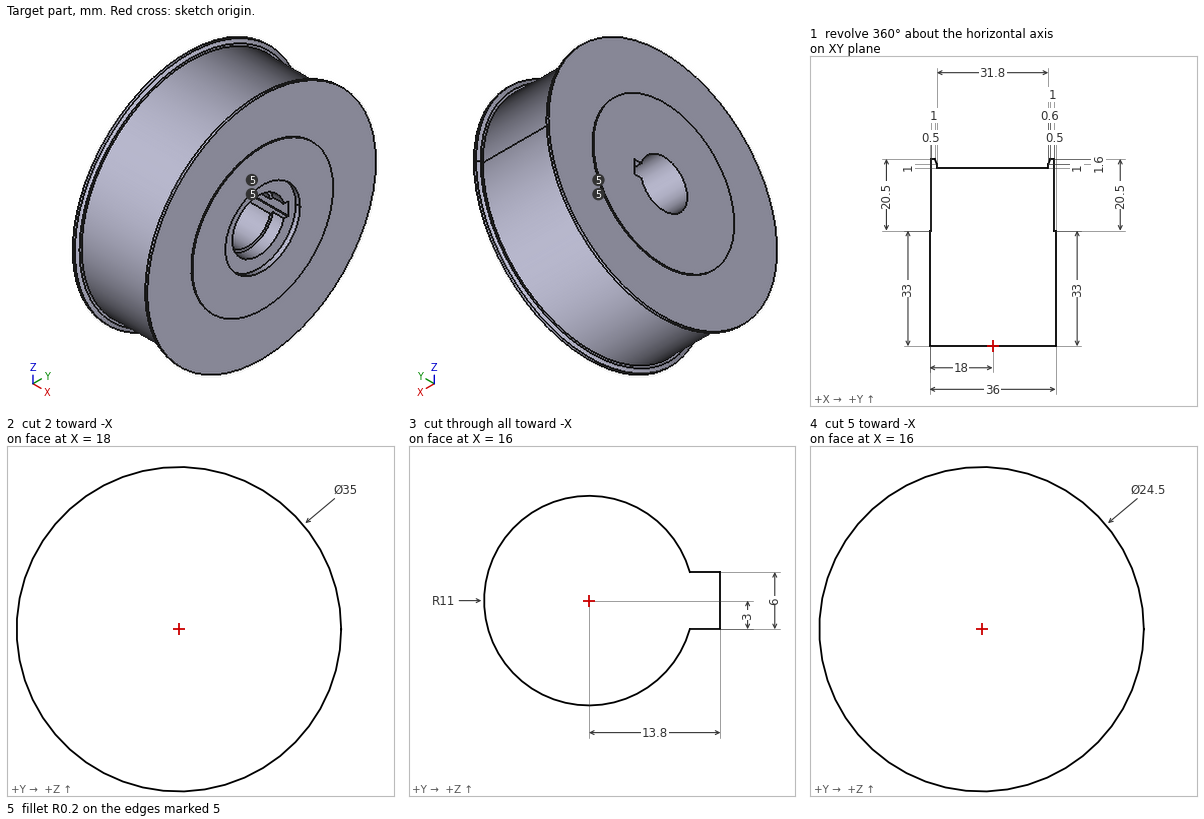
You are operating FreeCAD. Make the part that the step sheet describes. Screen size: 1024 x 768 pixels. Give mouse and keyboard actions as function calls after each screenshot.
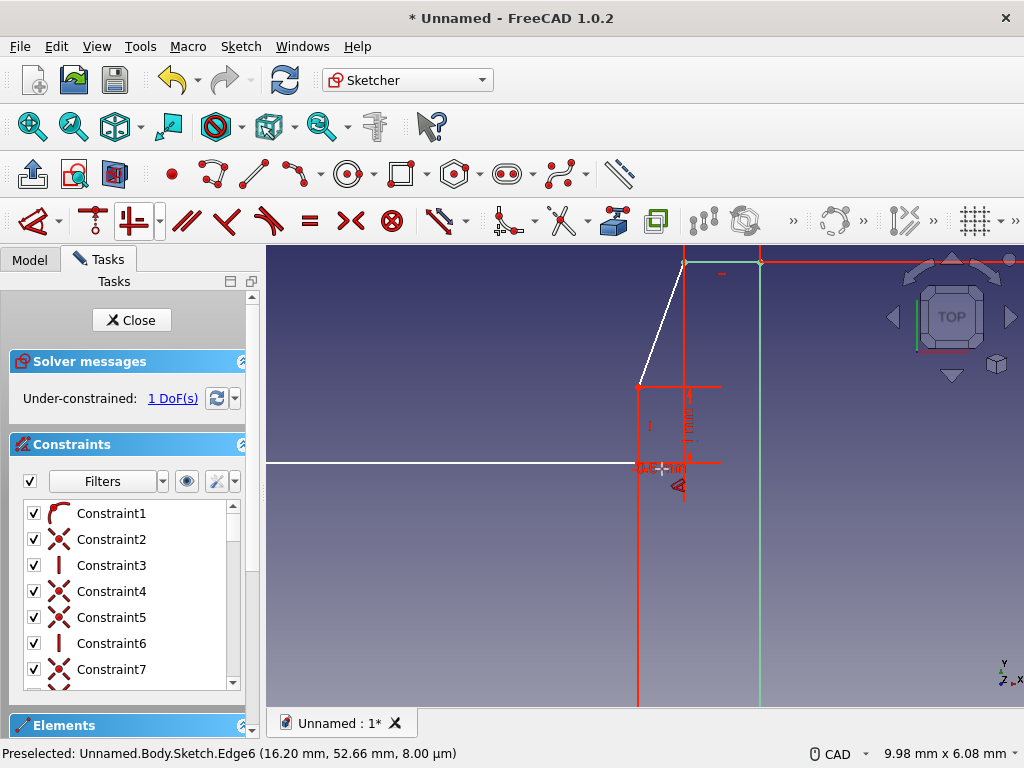
scroll(668, 330, down, 13)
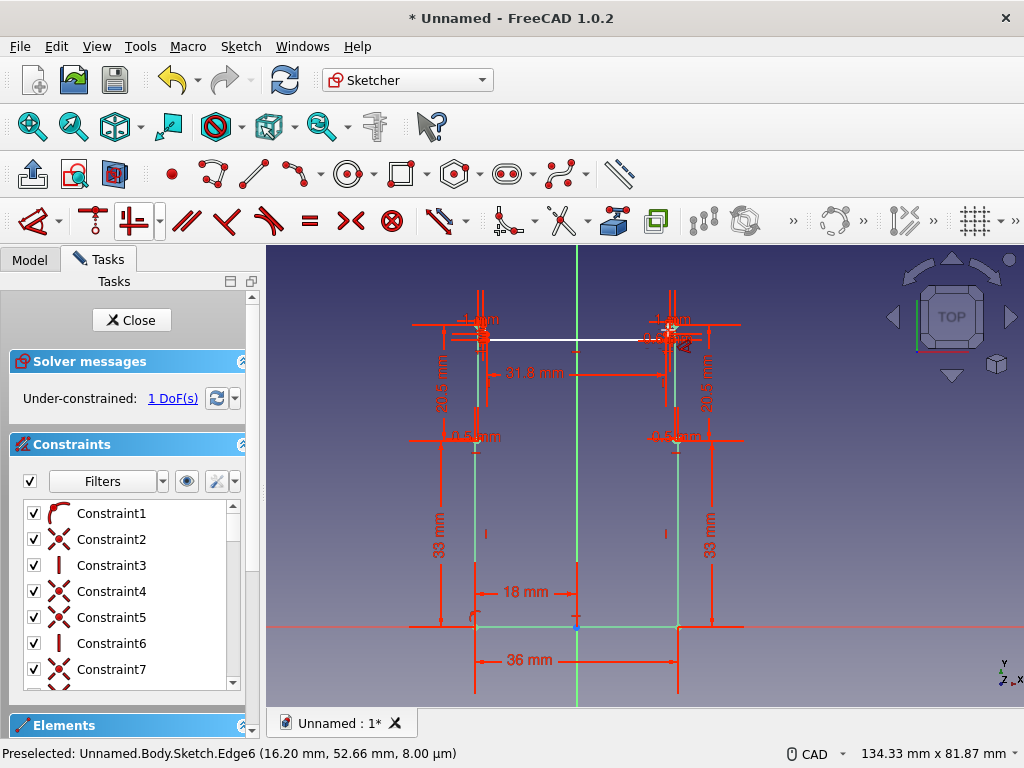
scroll(669, 328, up, 8)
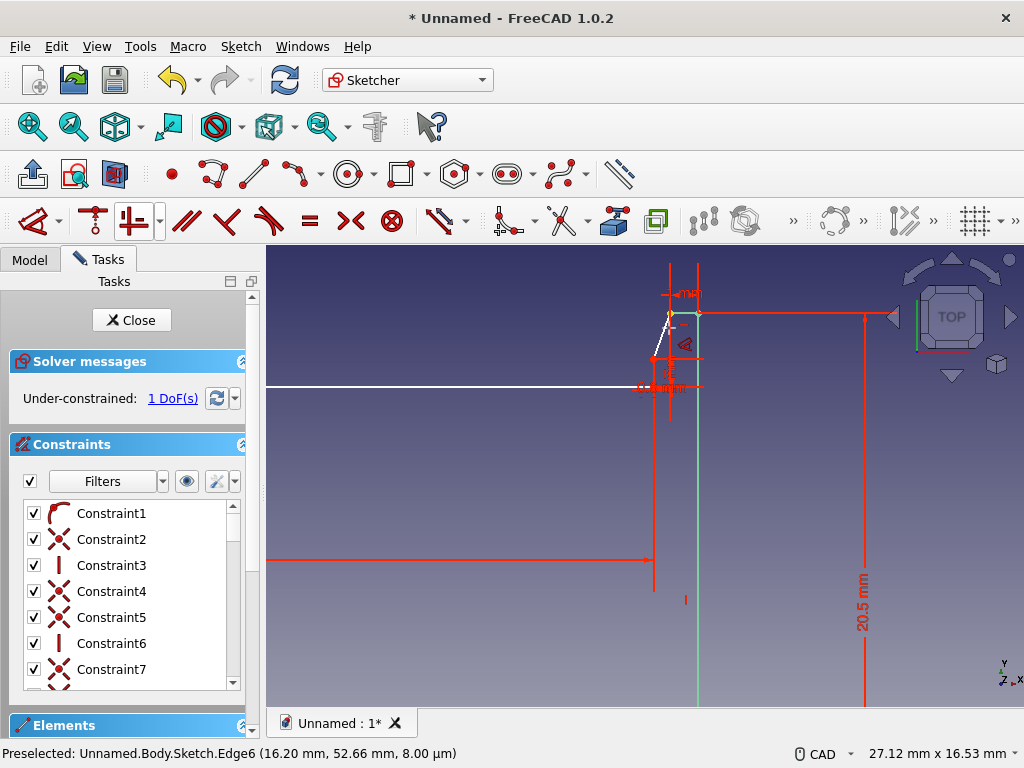
click(665, 327)
click(620, 336)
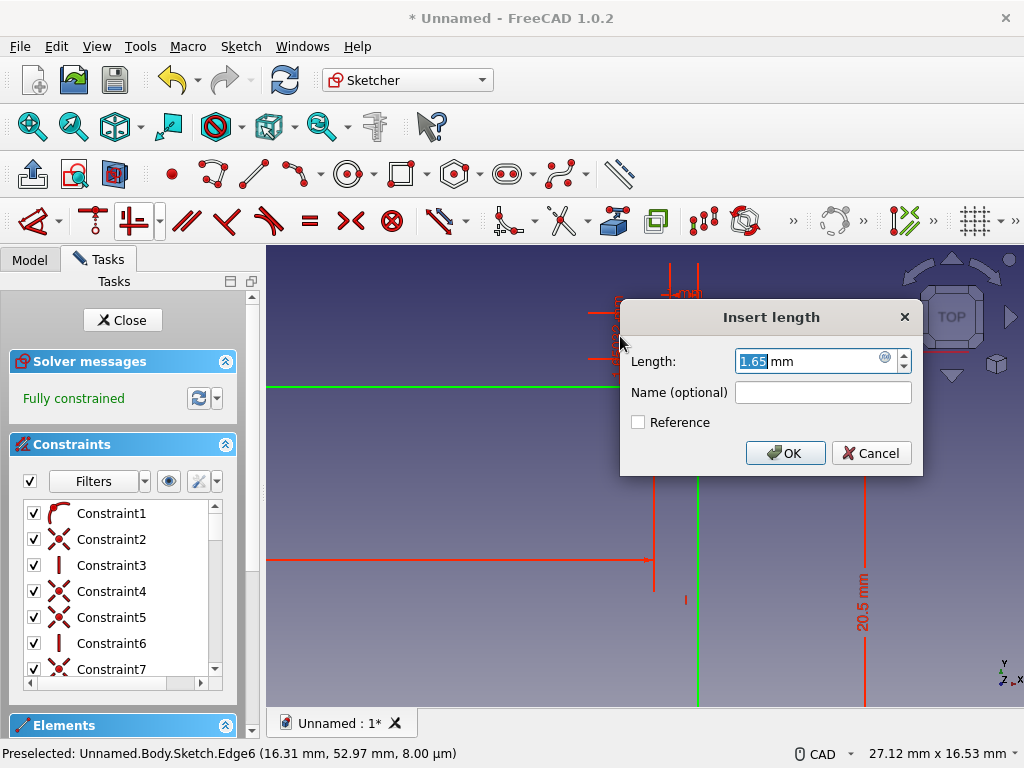
text(1.6)
key(Return)
key(Escape)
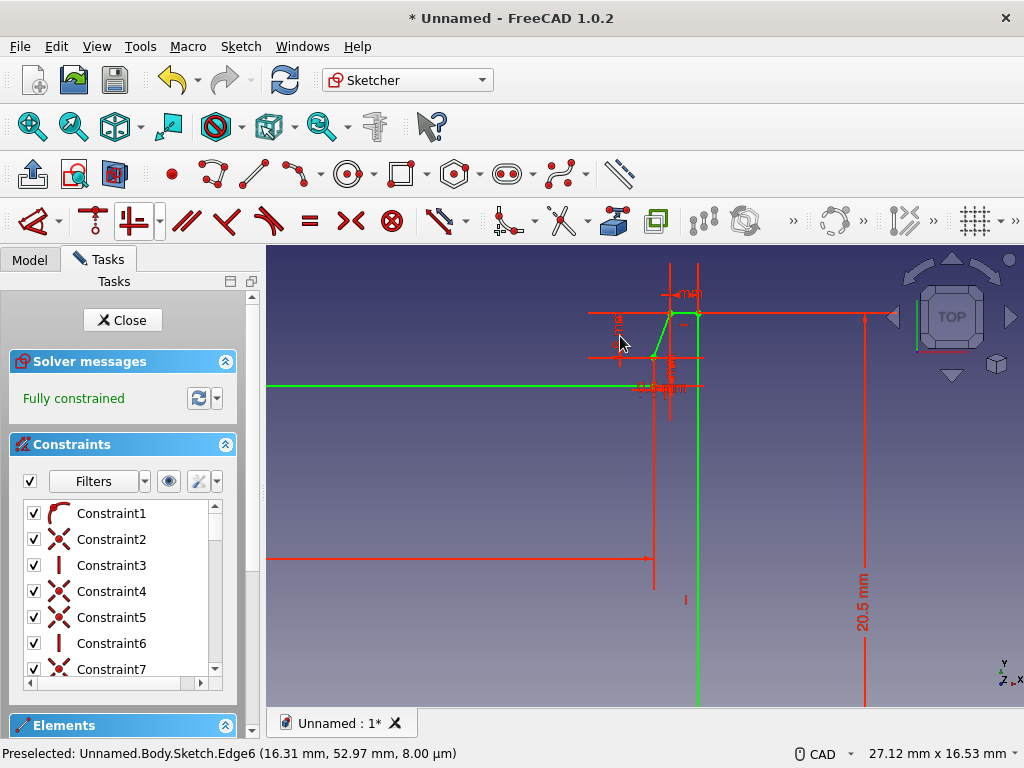
click(123, 320)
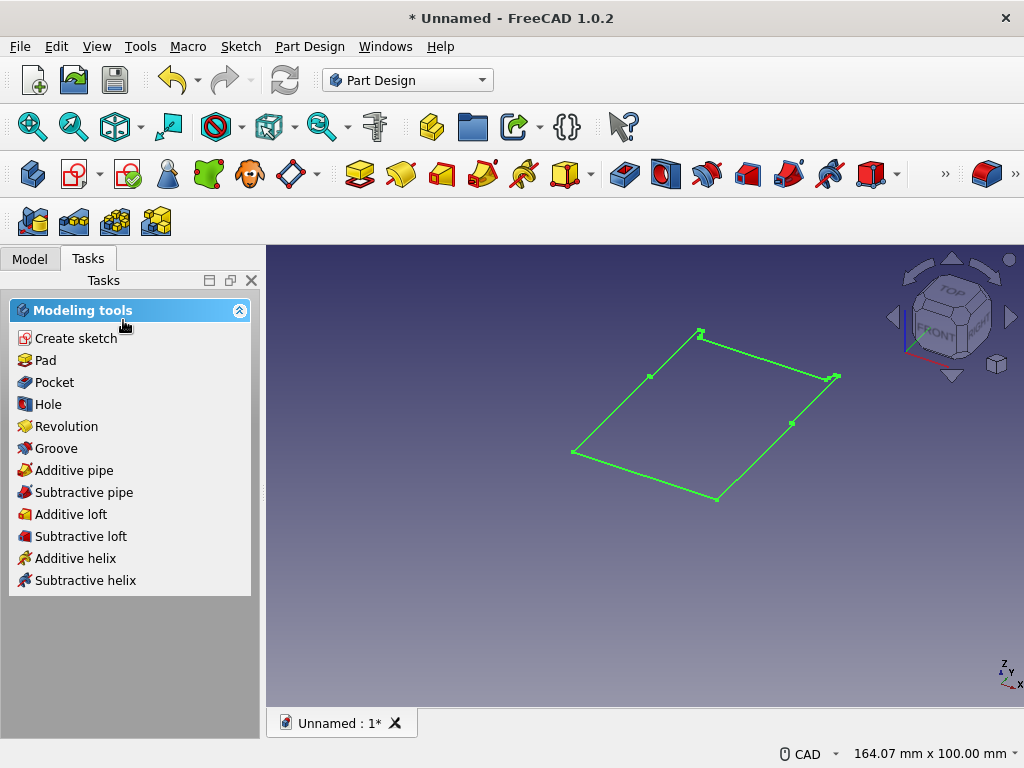
click(401, 174)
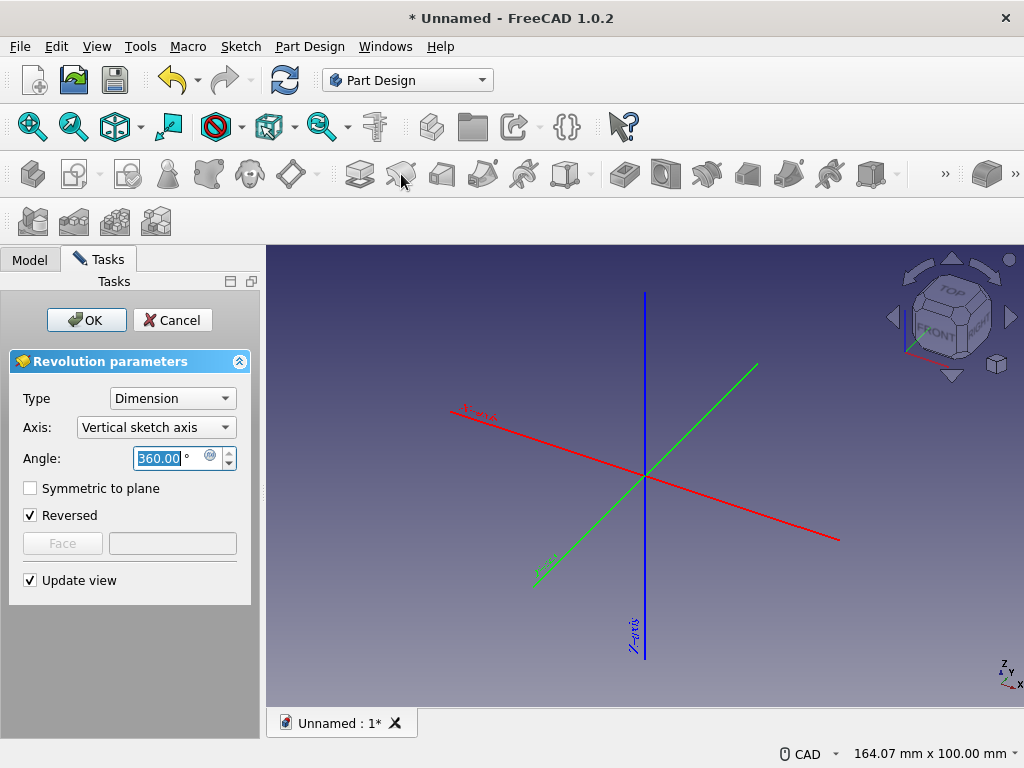
click(157, 428)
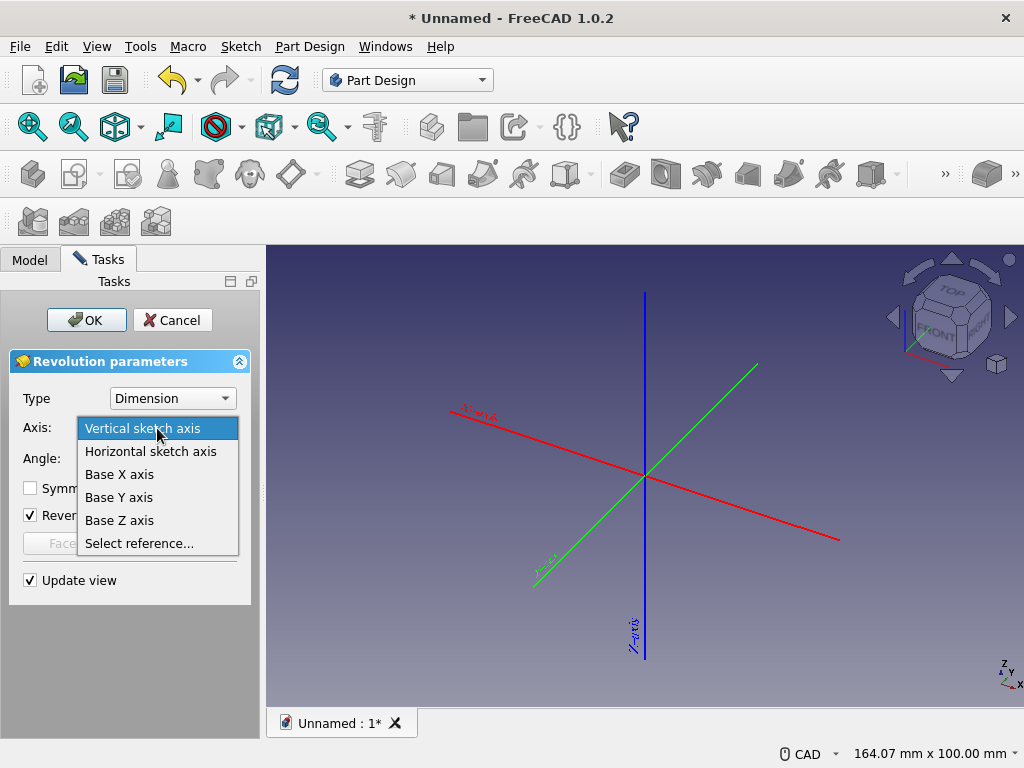
click(156, 452)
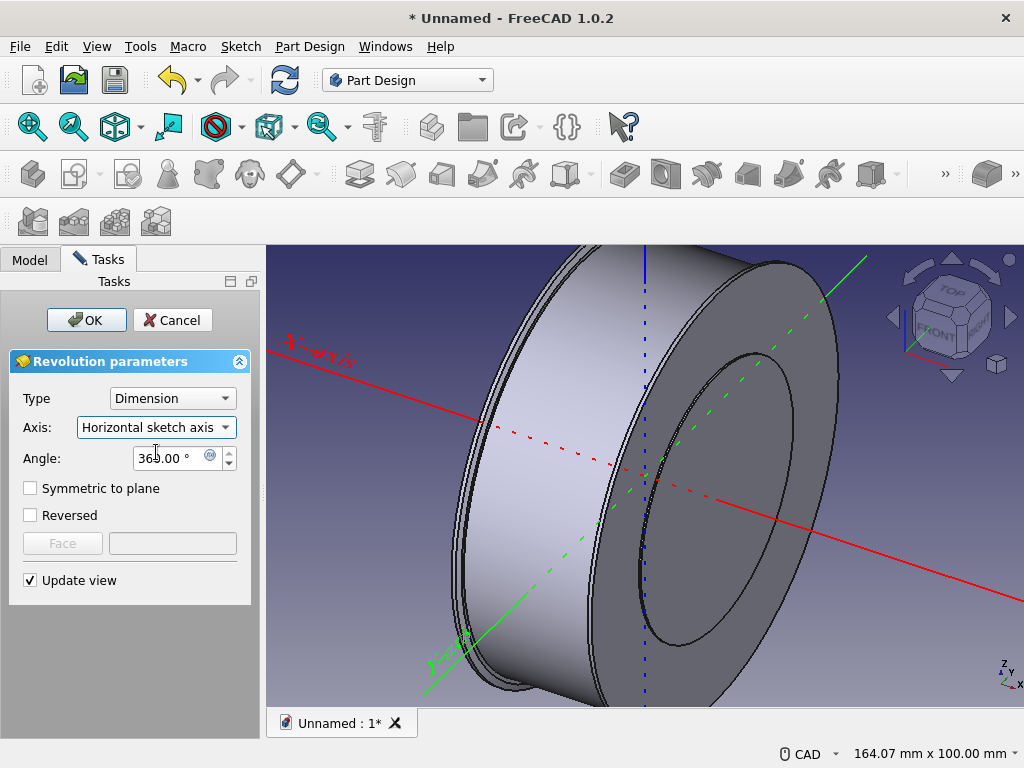
click(87, 320)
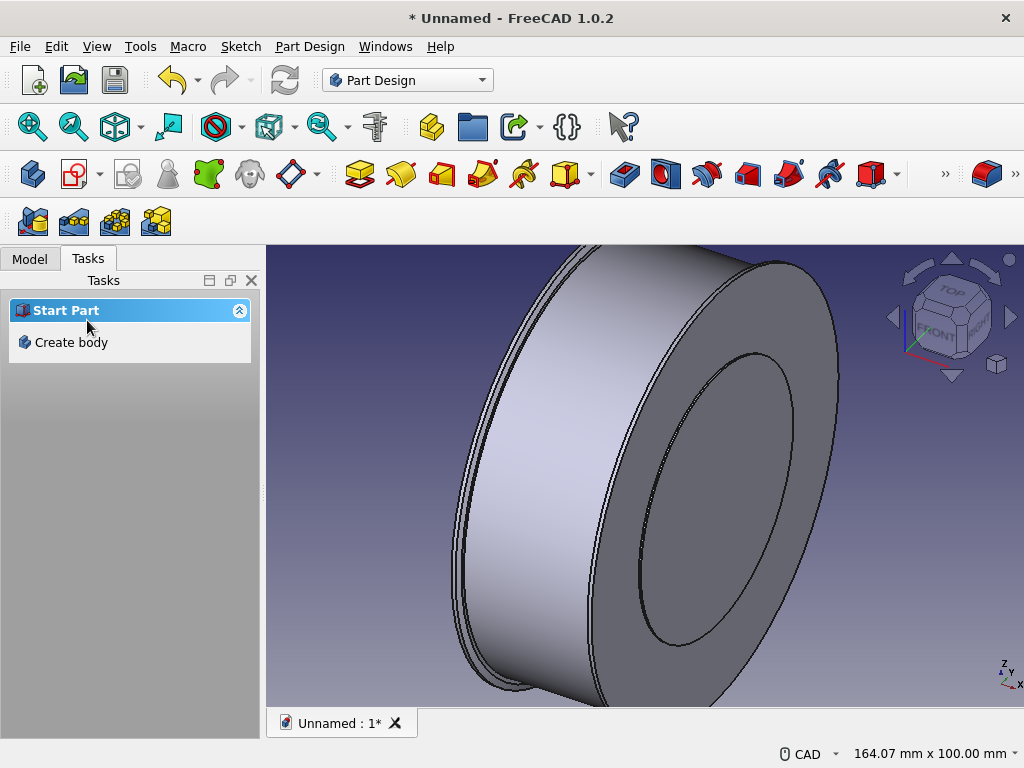
click(33, 128)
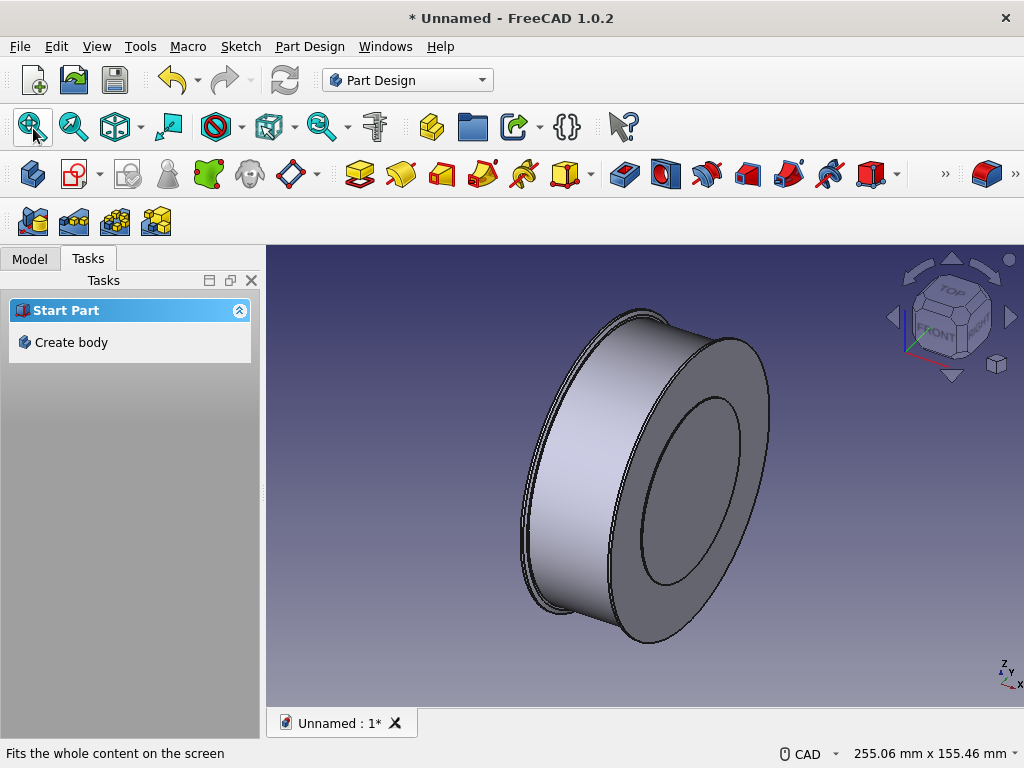
click(691, 490)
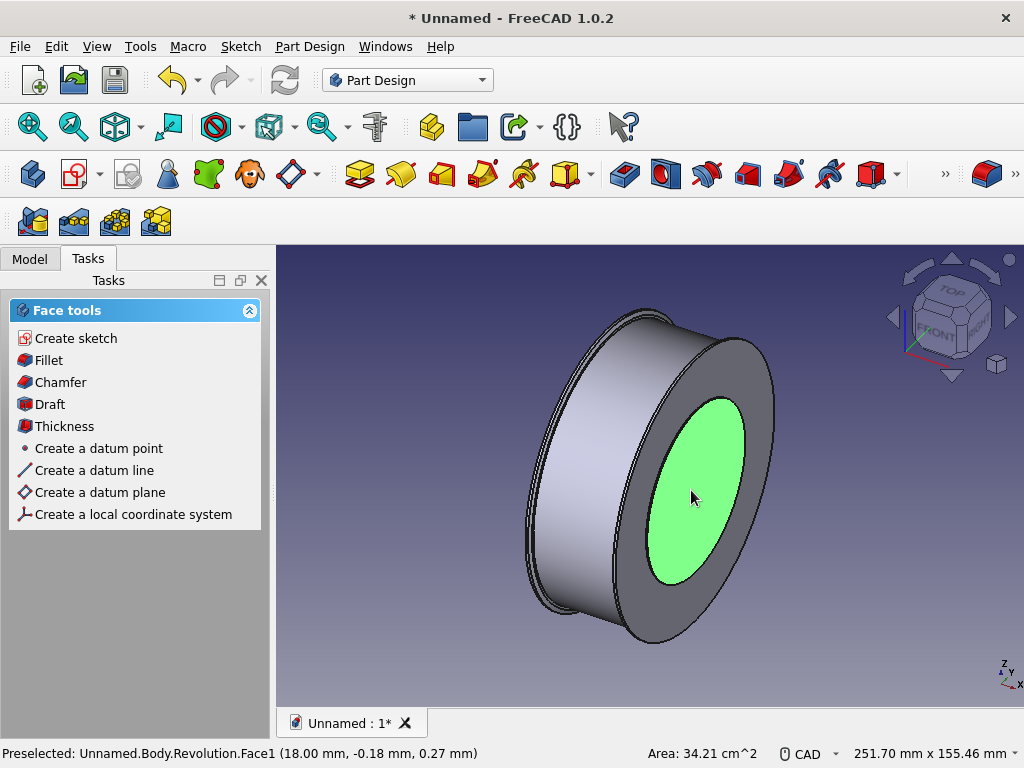
click(74, 174)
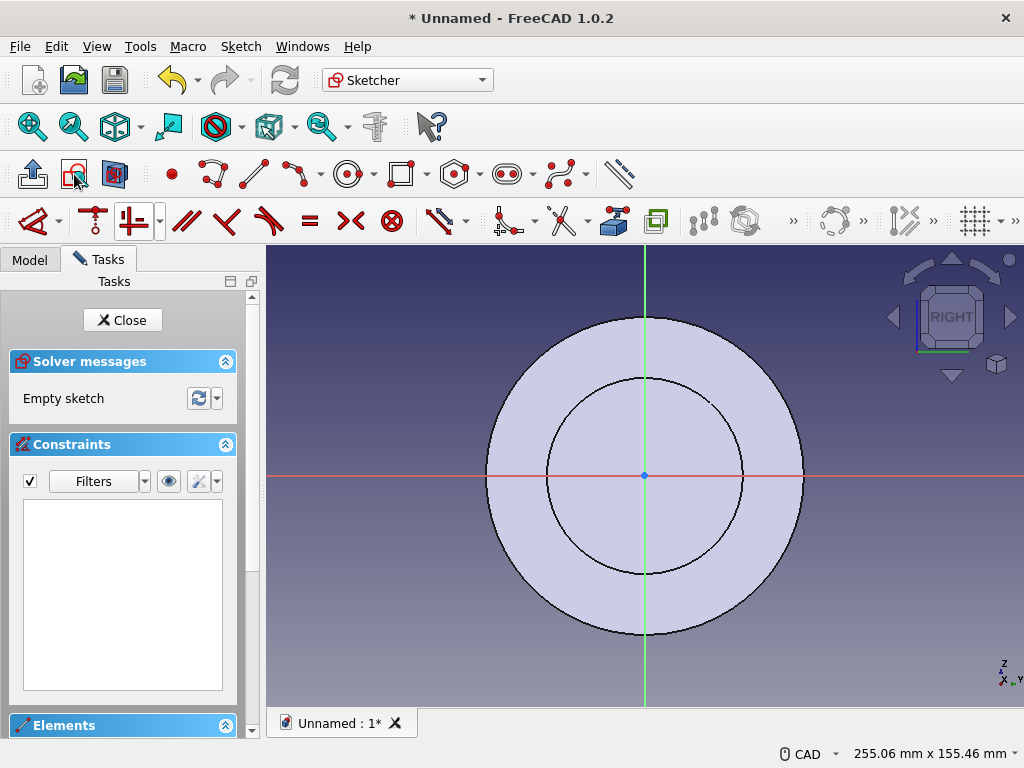
scroll(685, 476, up, 5)